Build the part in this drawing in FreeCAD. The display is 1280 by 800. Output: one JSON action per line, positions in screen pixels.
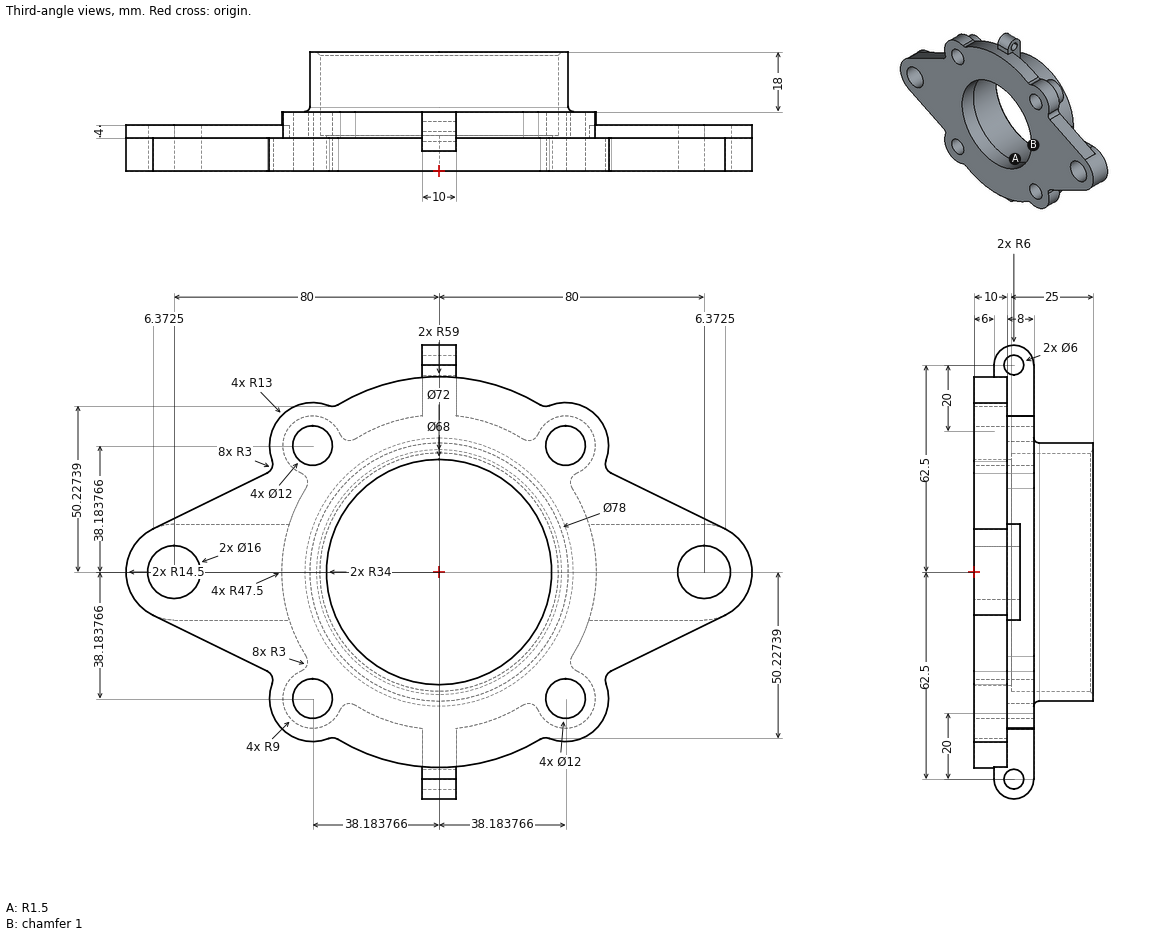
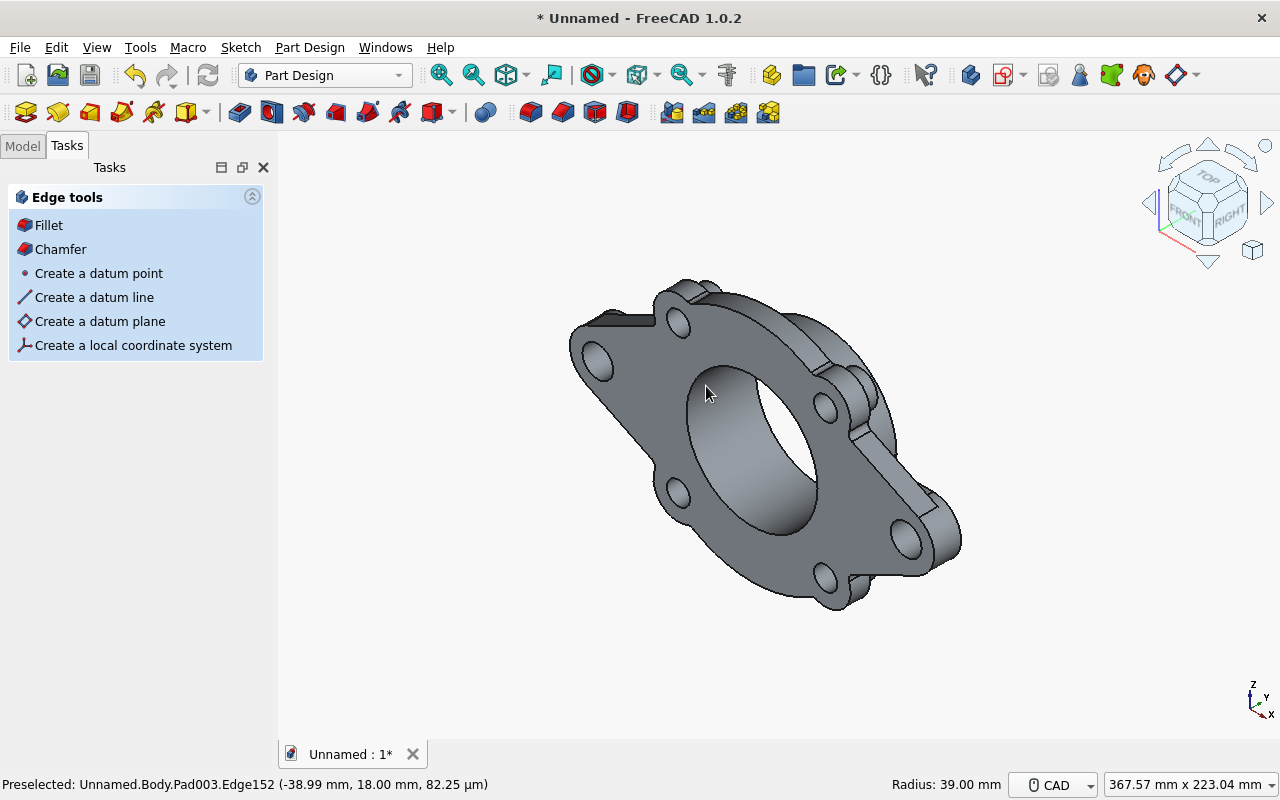
{"action": "left_click", "coordinate": [532, 112]}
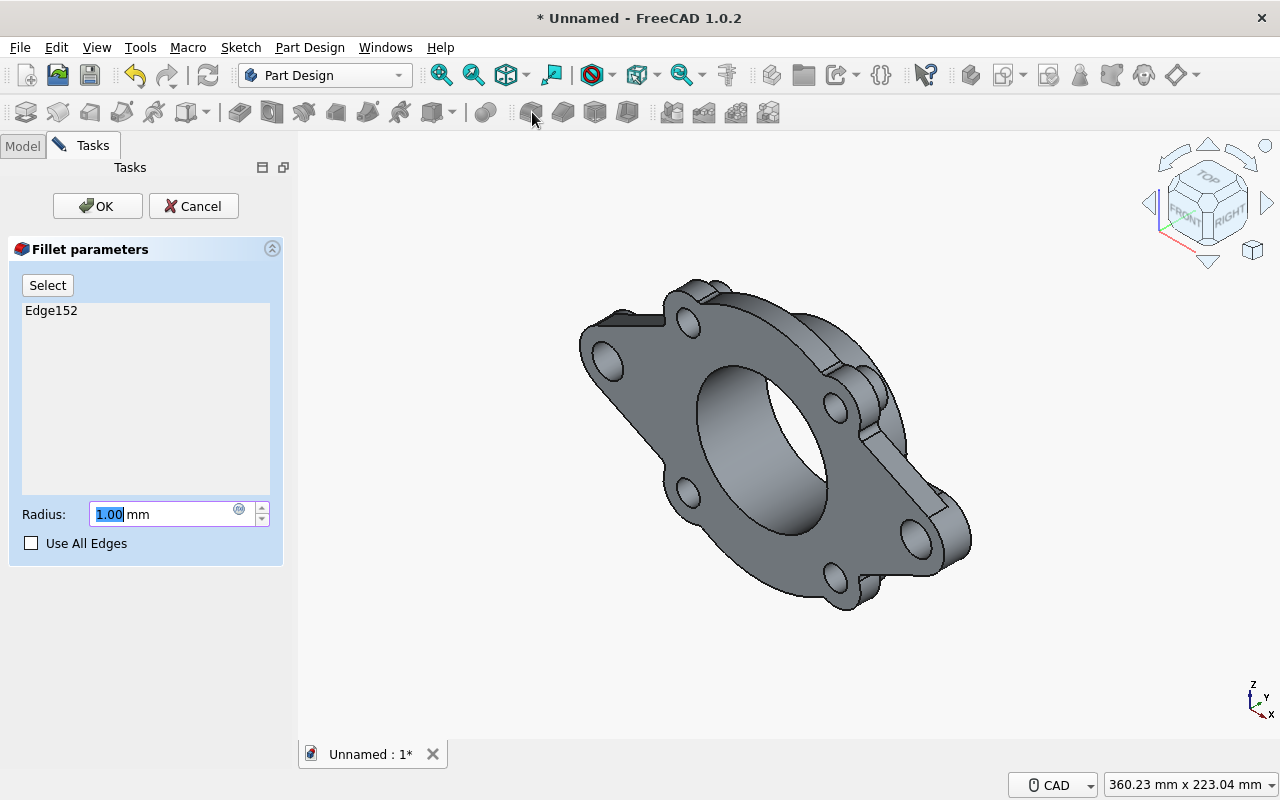
{"action": "type", "text": "1.5"}
{"action": "key", "text": "Tab"}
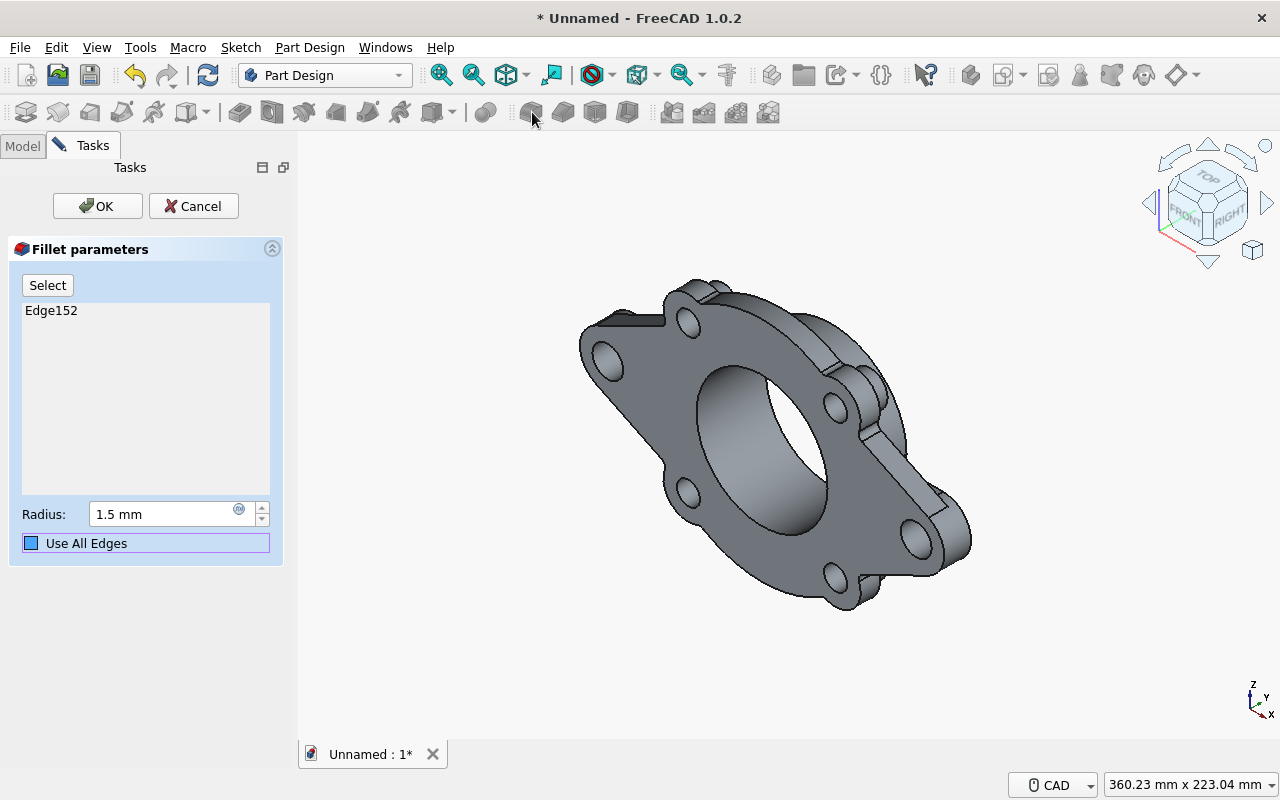
{"action": "left_click", "coordinate": [98, 206]}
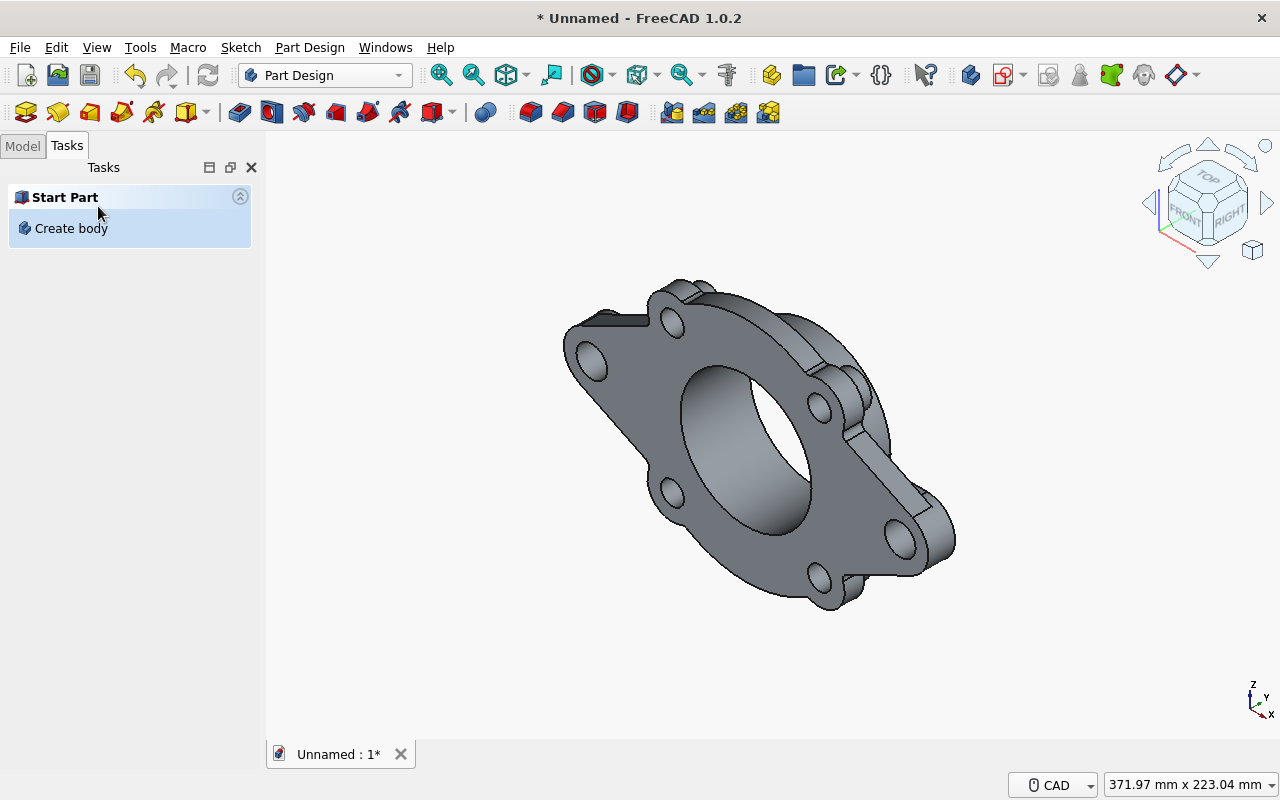
{"action": "key", "text": "4"}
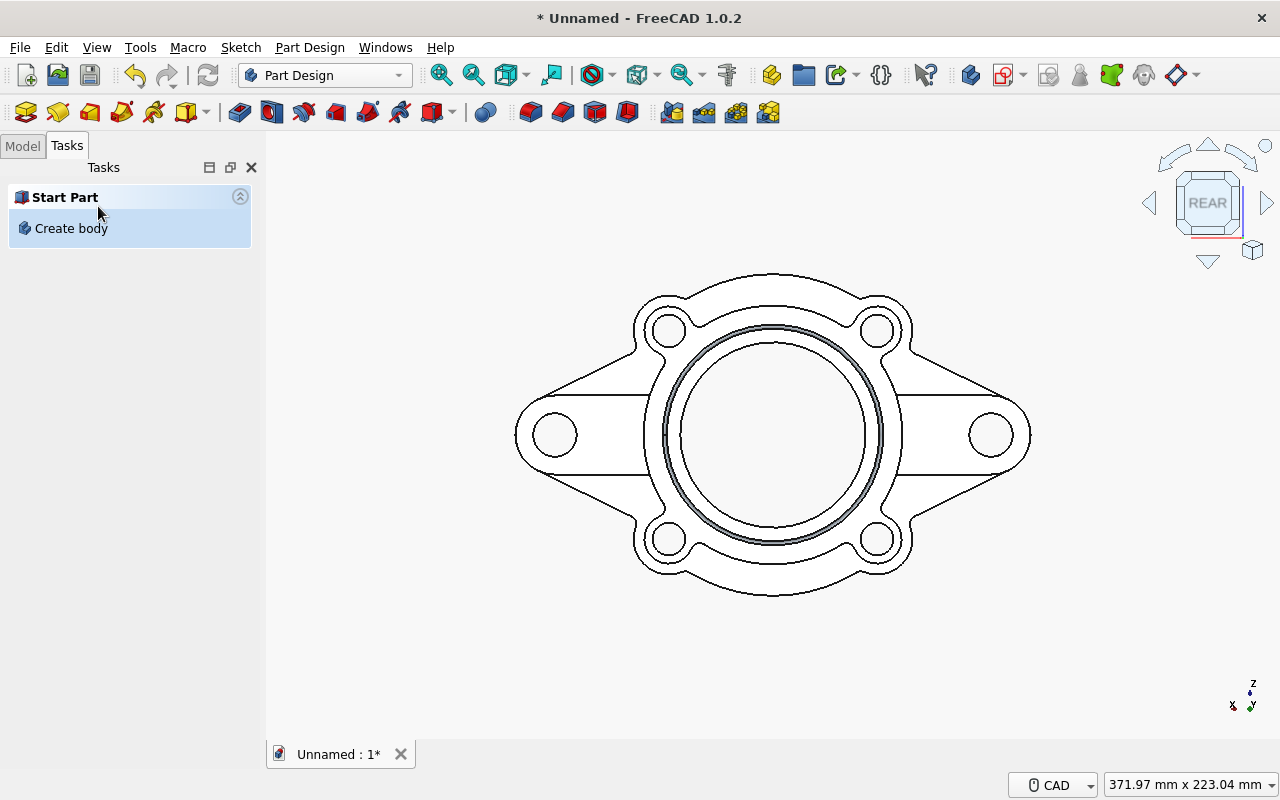
{"action": "scroll", "coordinate": [743, 343], "scroll_direction": "up", "scroll_amount": 7}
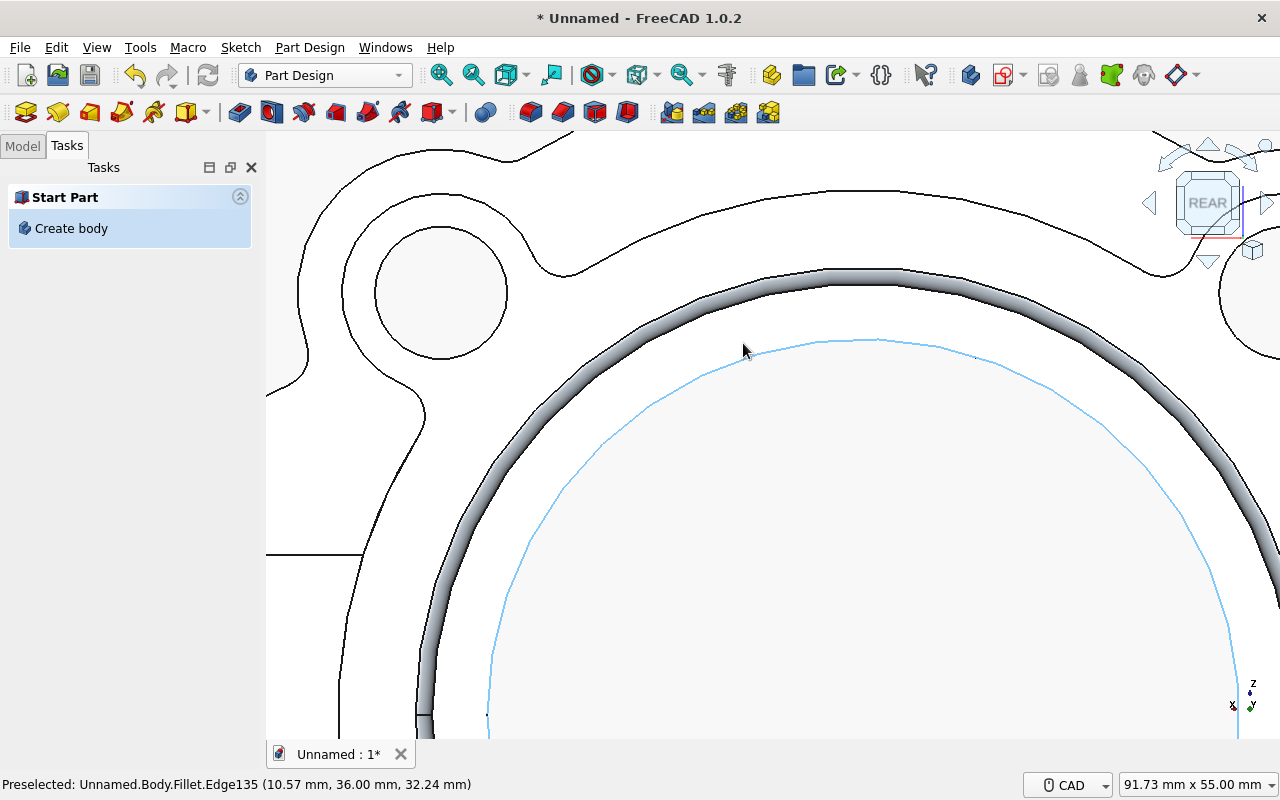
{"action": "left_click", "coordinate": [740, 344]}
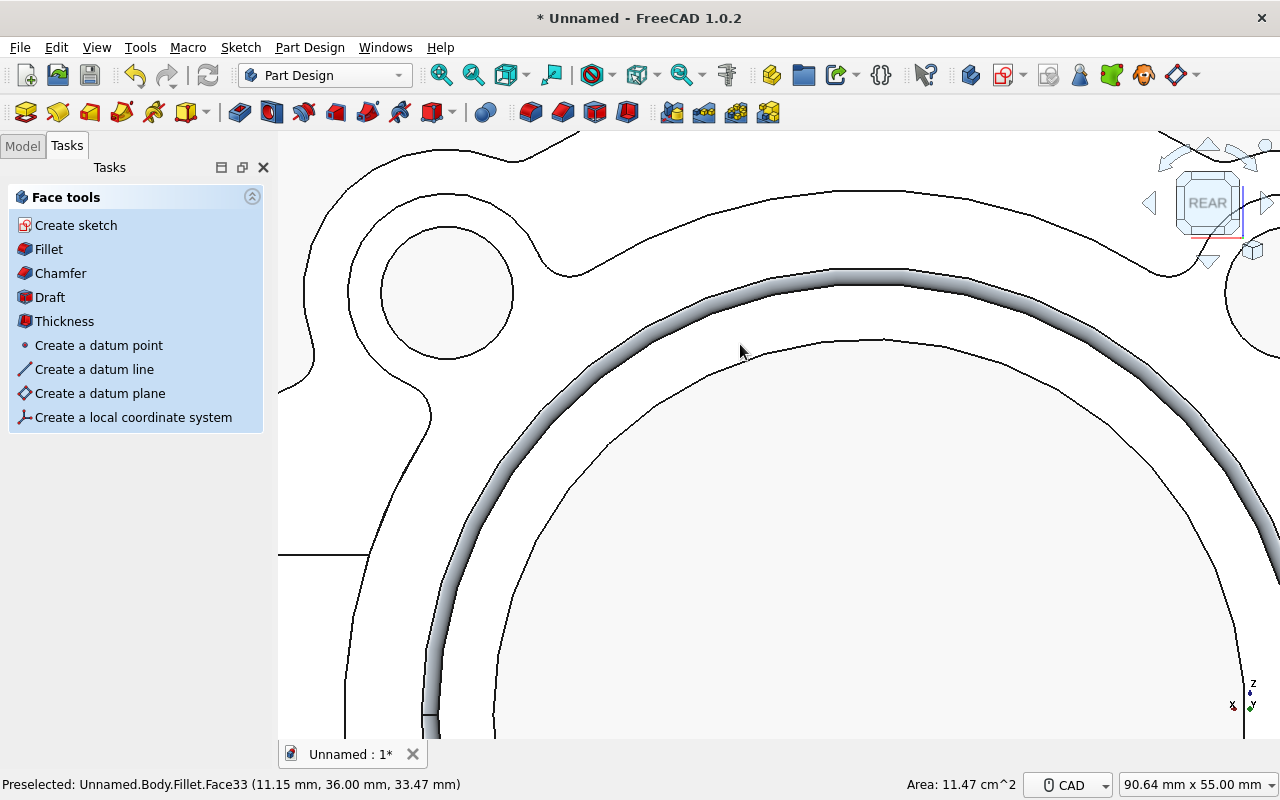
{"action": "left_click", "coordinate": [1004, 76]}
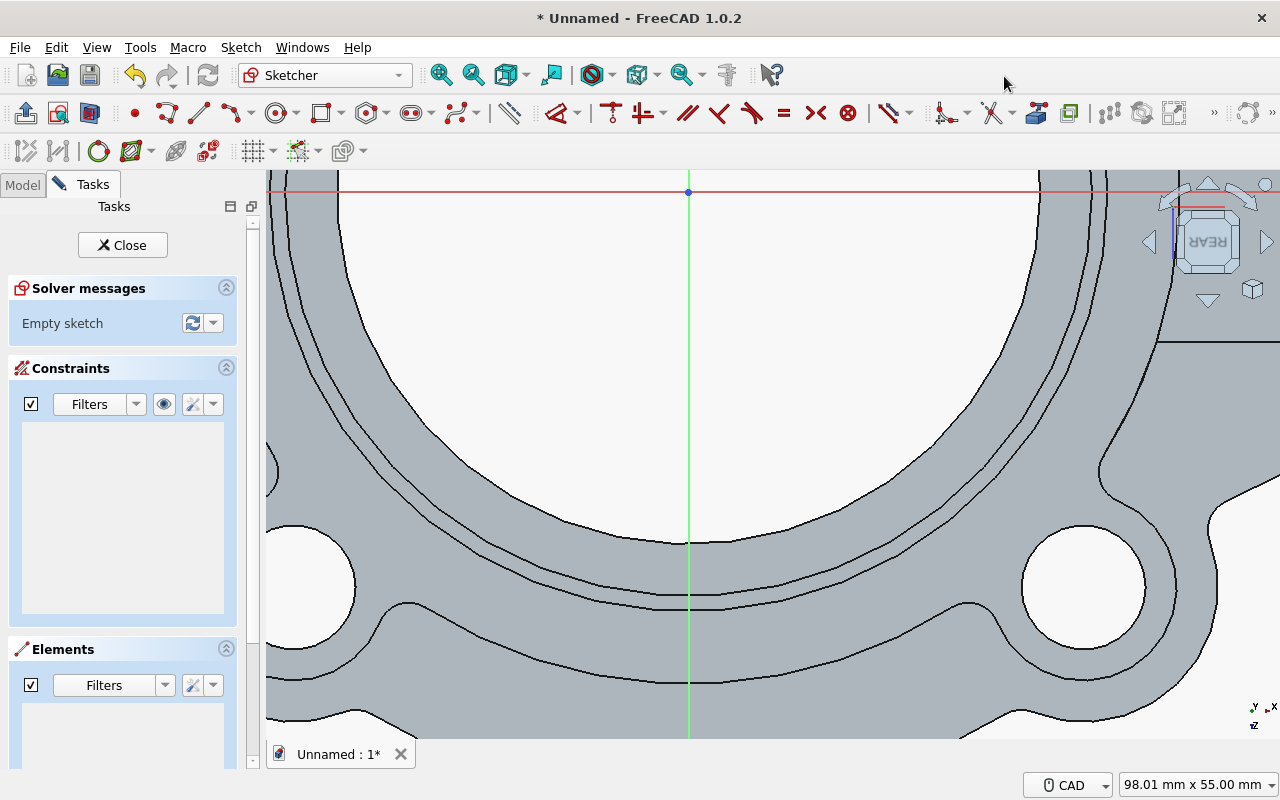
{"action": "scroll", "coordinate": [717, 668], "scroll_direction": "down", "scroll_amount": 4}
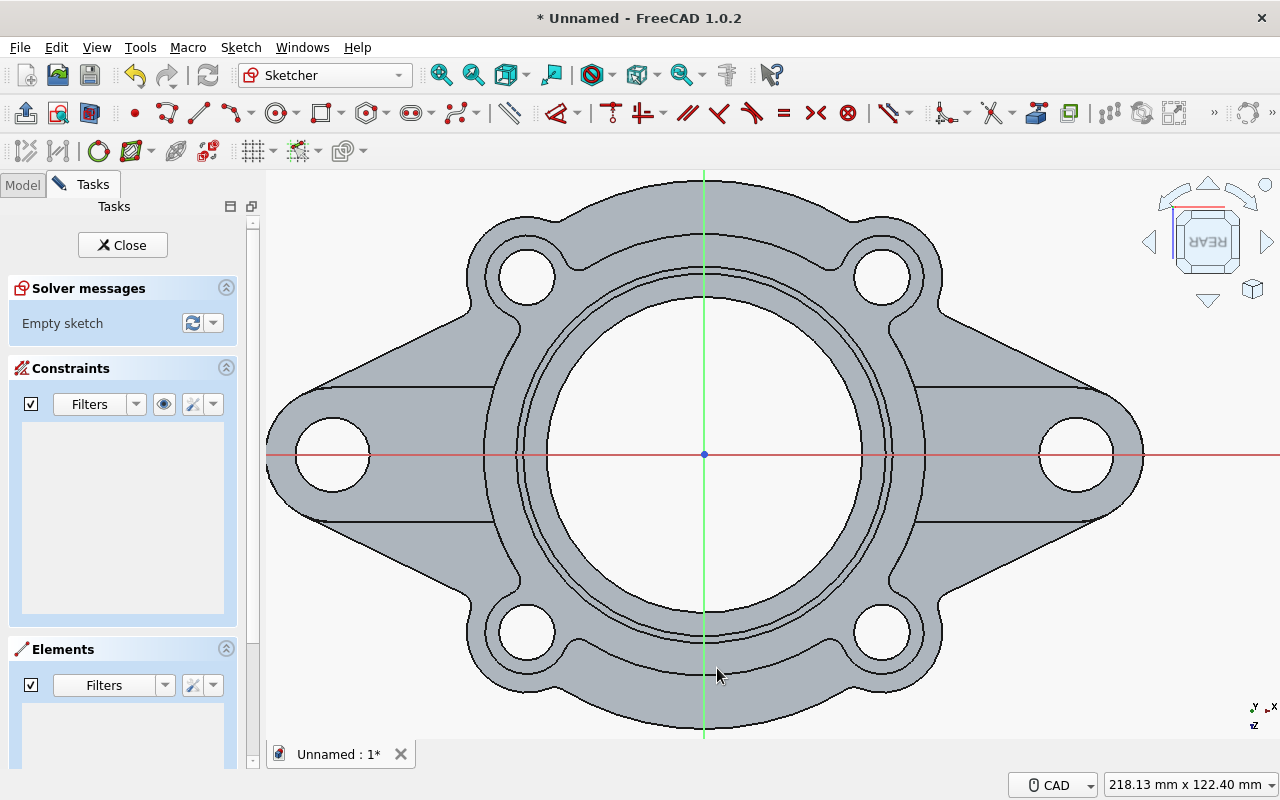
{"action": "left_click", "coordinate": [276, 114]}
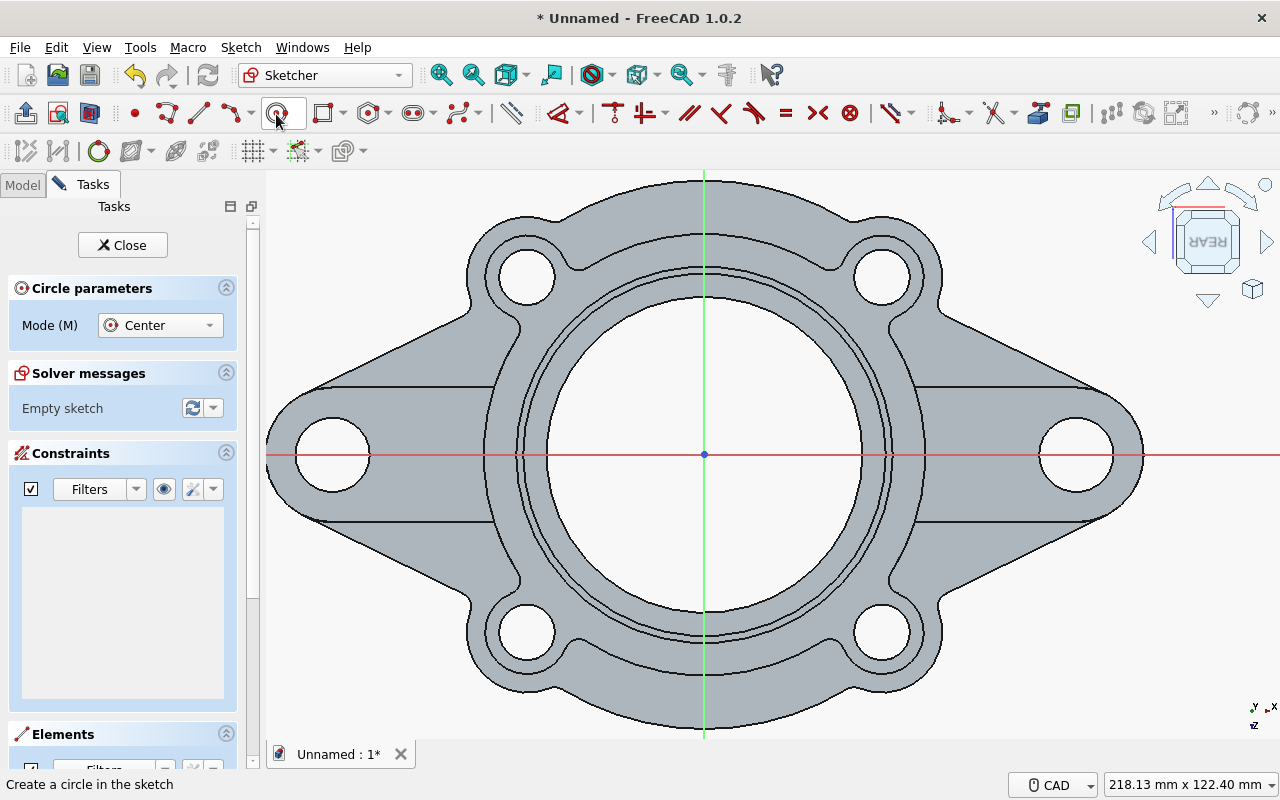
{"action": "left_click", "coordinate": [704, 455]}
{"action": "mouse_move", "coordinate": [823, 336]}